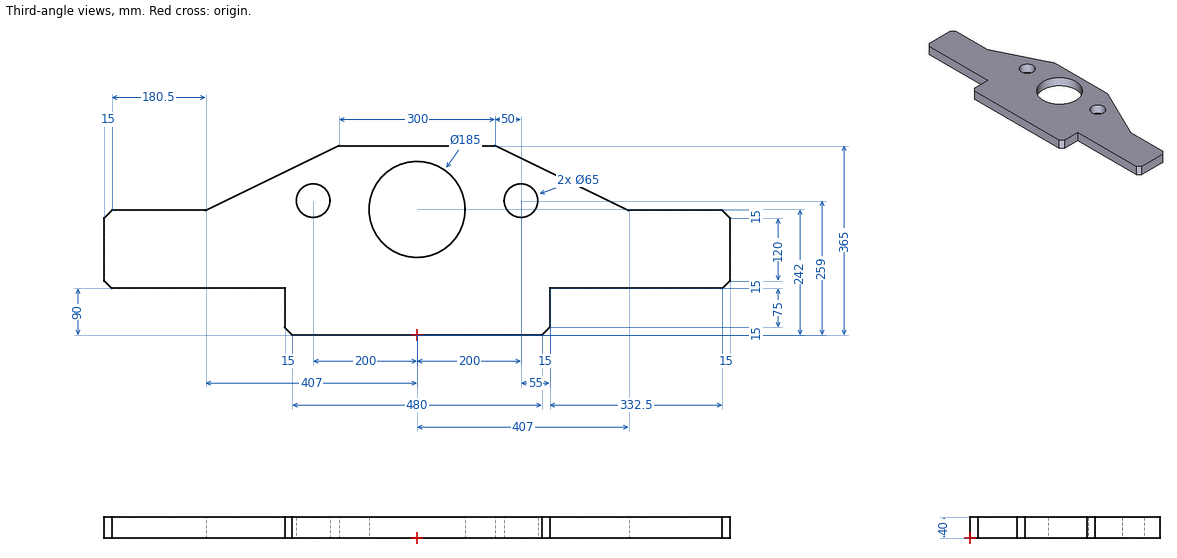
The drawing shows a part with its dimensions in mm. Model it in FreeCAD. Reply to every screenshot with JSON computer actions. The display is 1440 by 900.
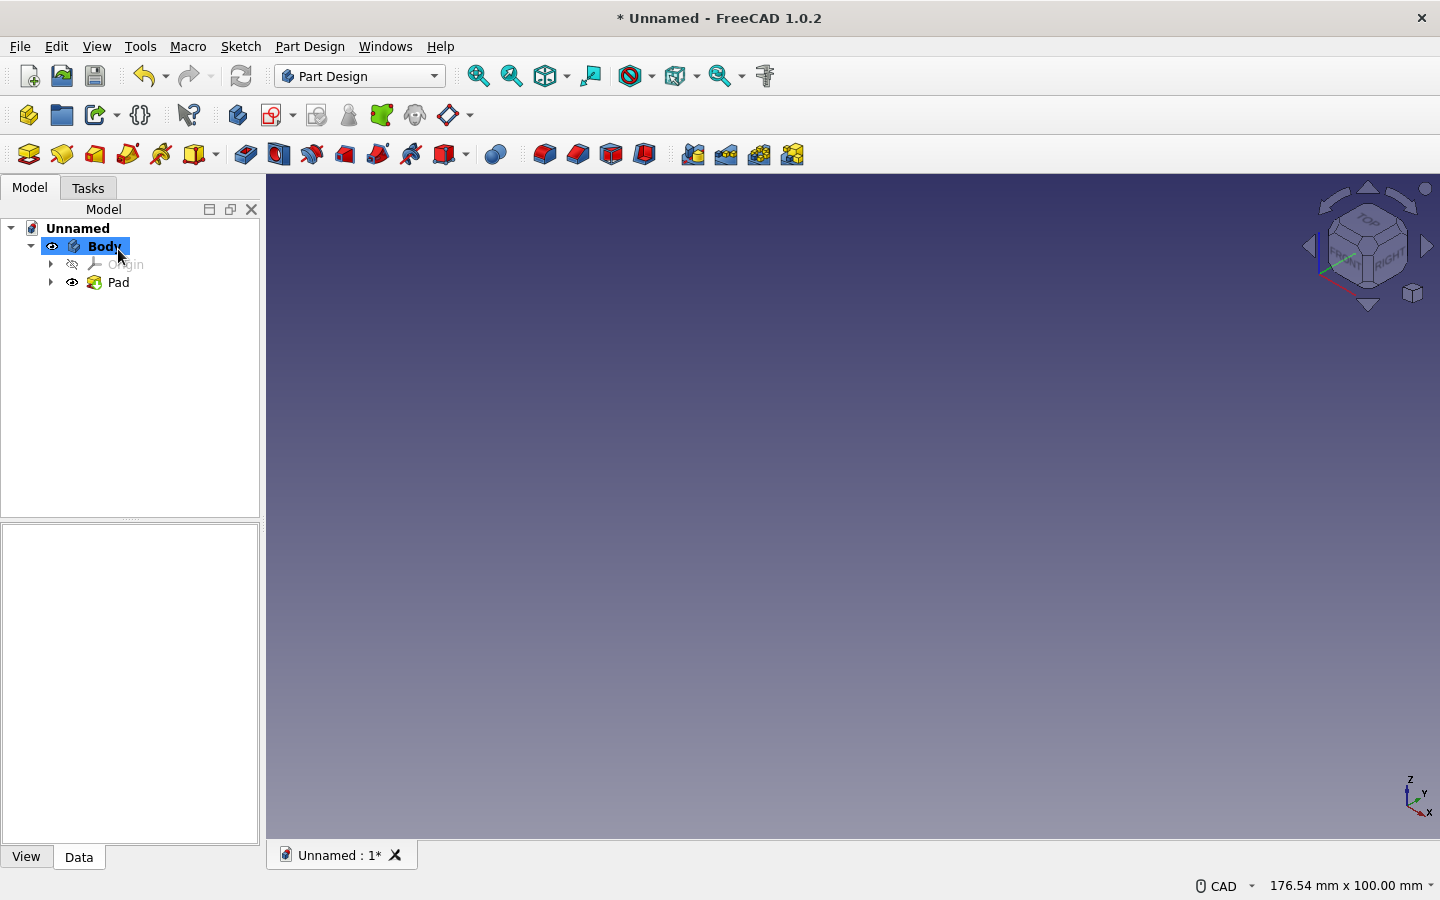
{"action": "left_click", "coordinate": [479, 76]}